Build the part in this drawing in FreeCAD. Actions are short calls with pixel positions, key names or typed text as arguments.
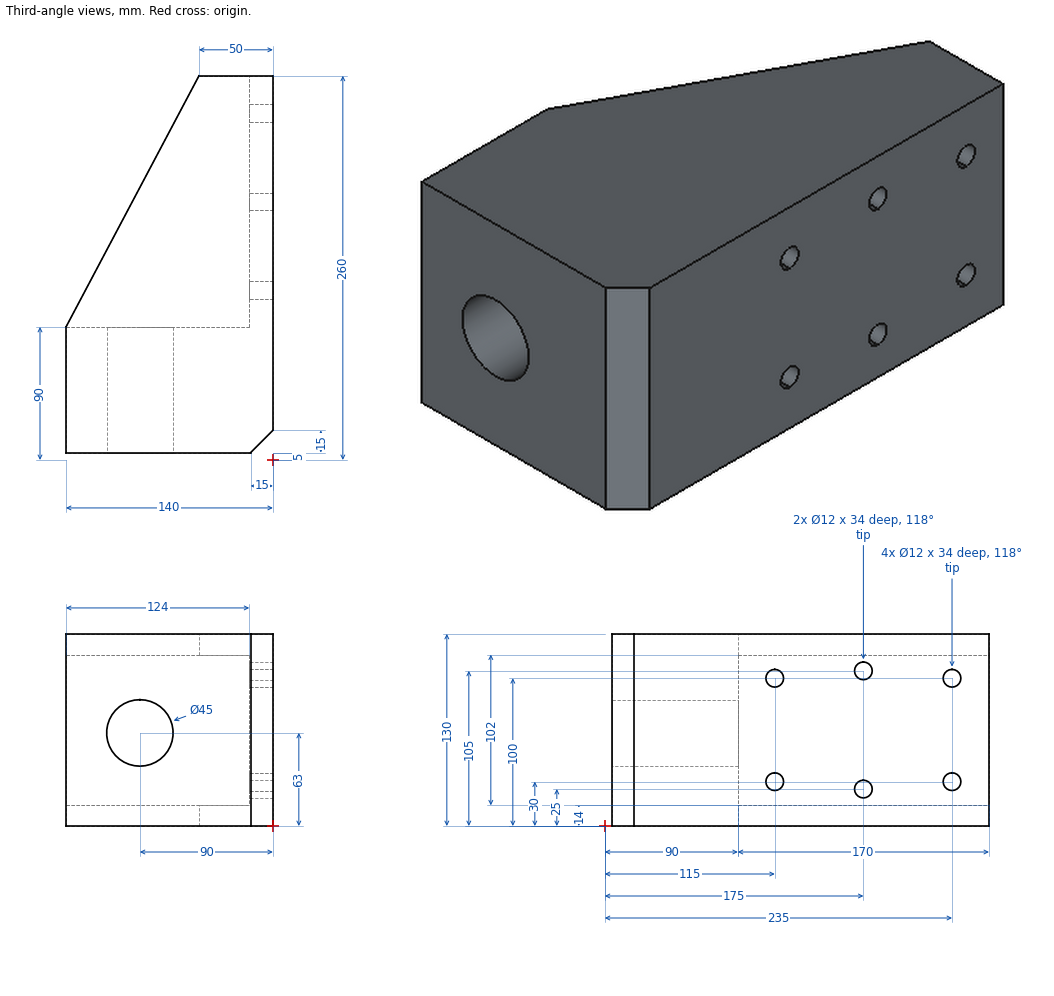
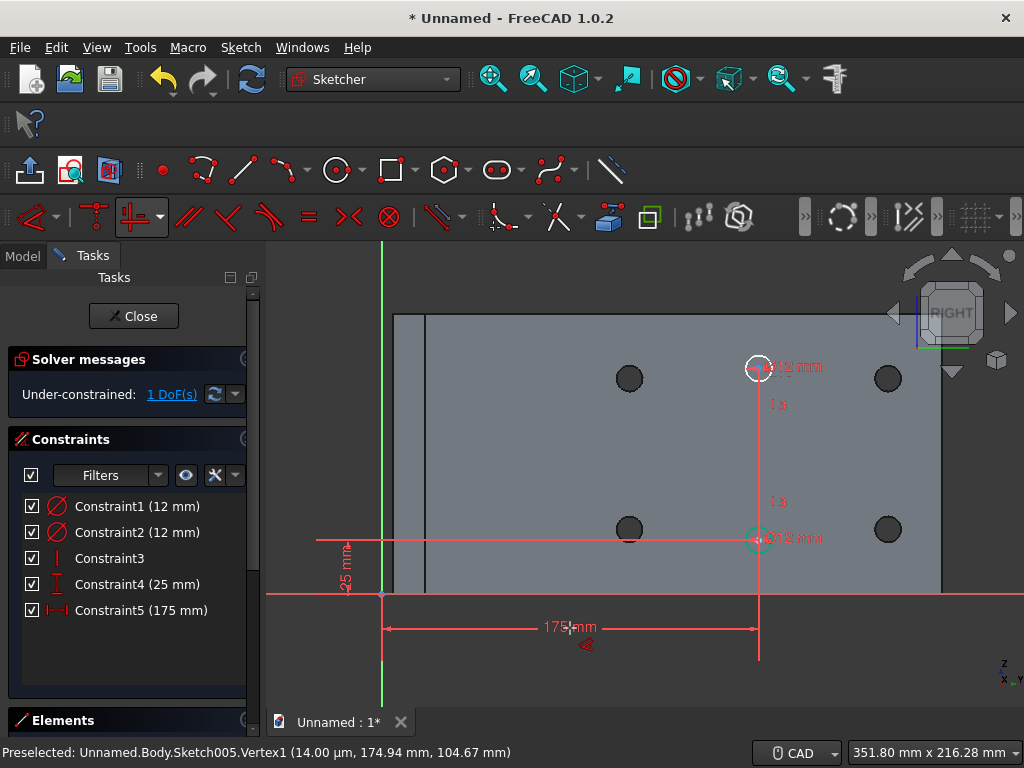
click(759, 369)
click(348, 481)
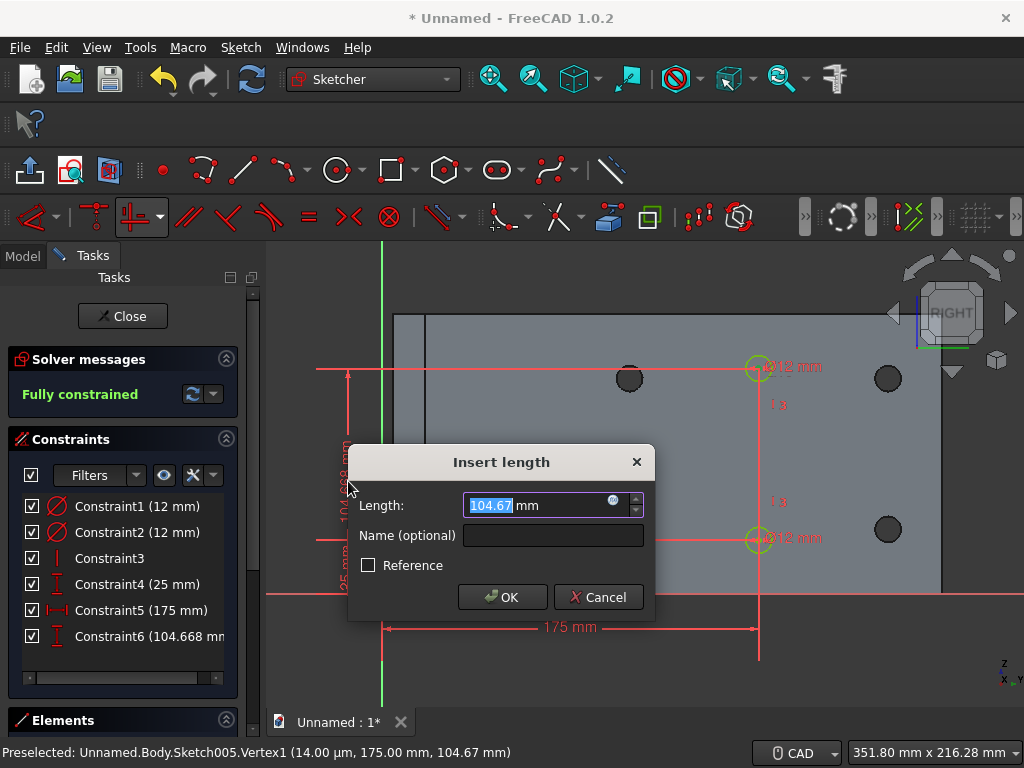
text(105)
key(Return)
key(Escape)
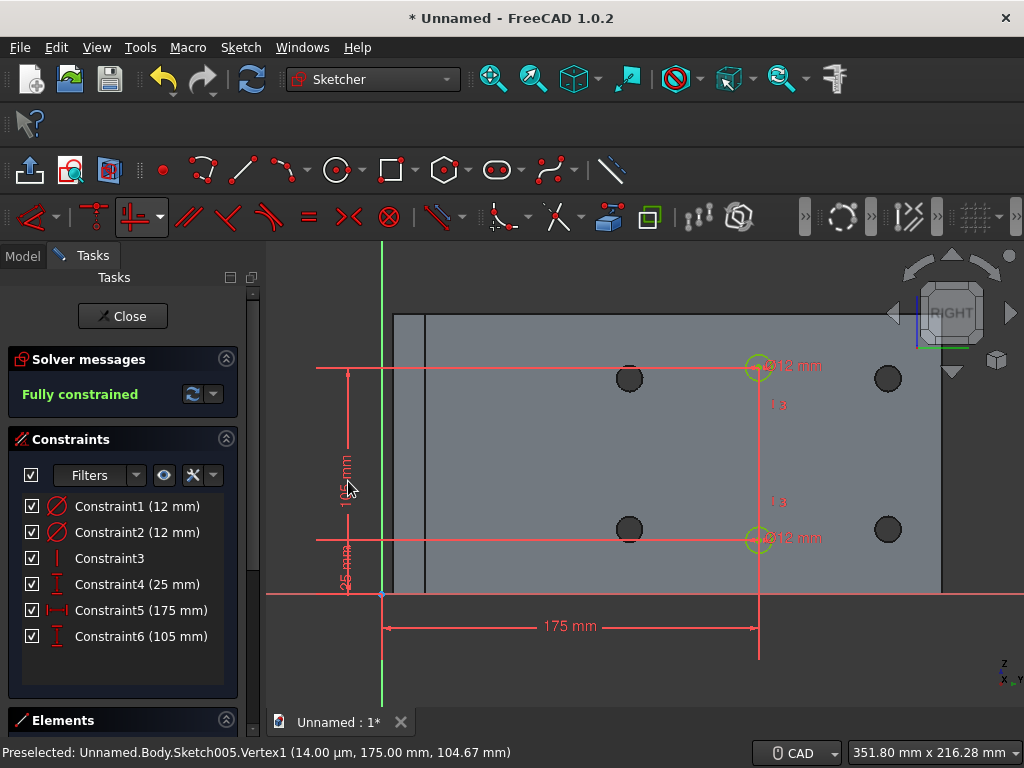
click(123, 316)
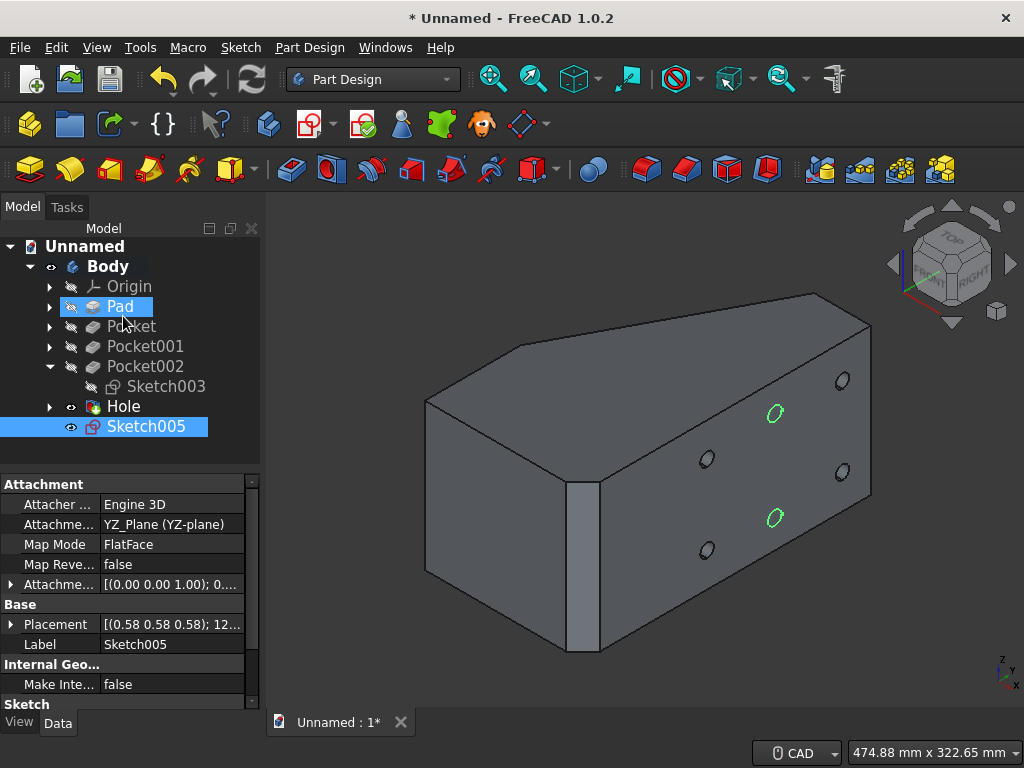
click(332, 170)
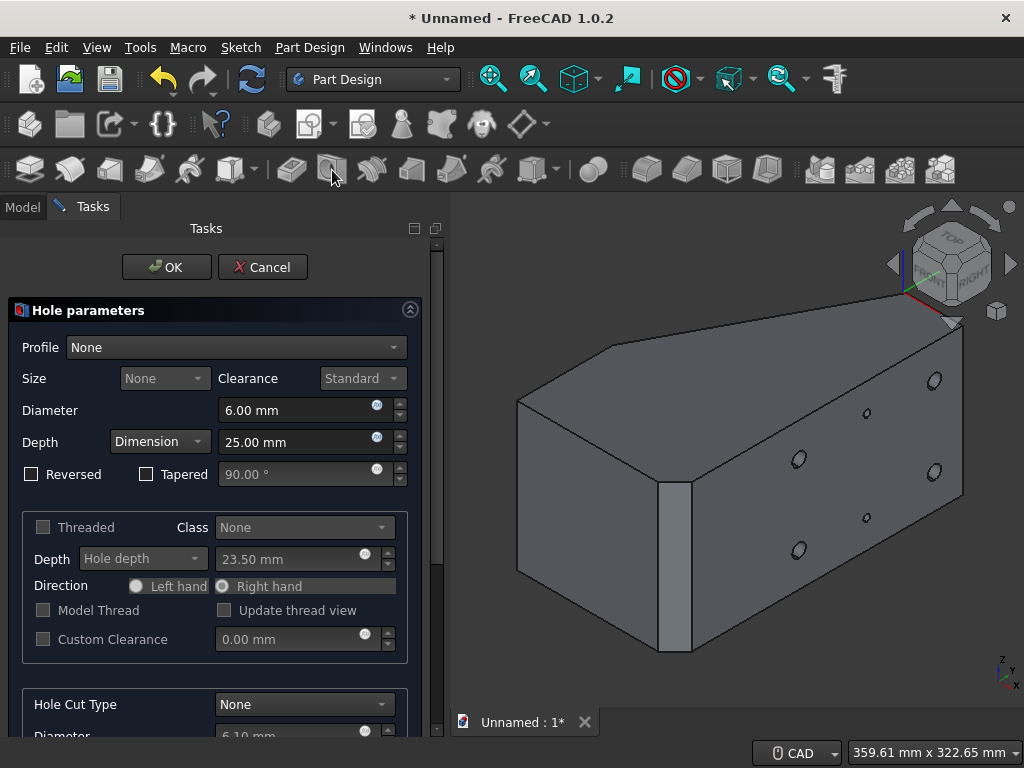
triple_click(305, 410)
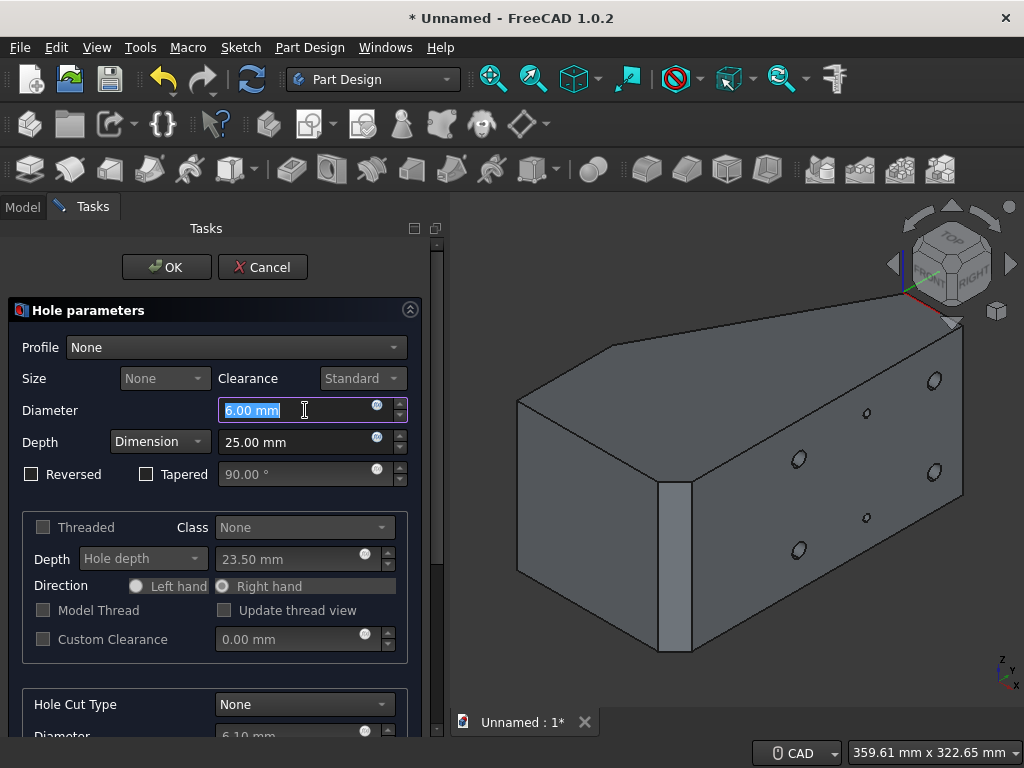
text(12)
key(Tab)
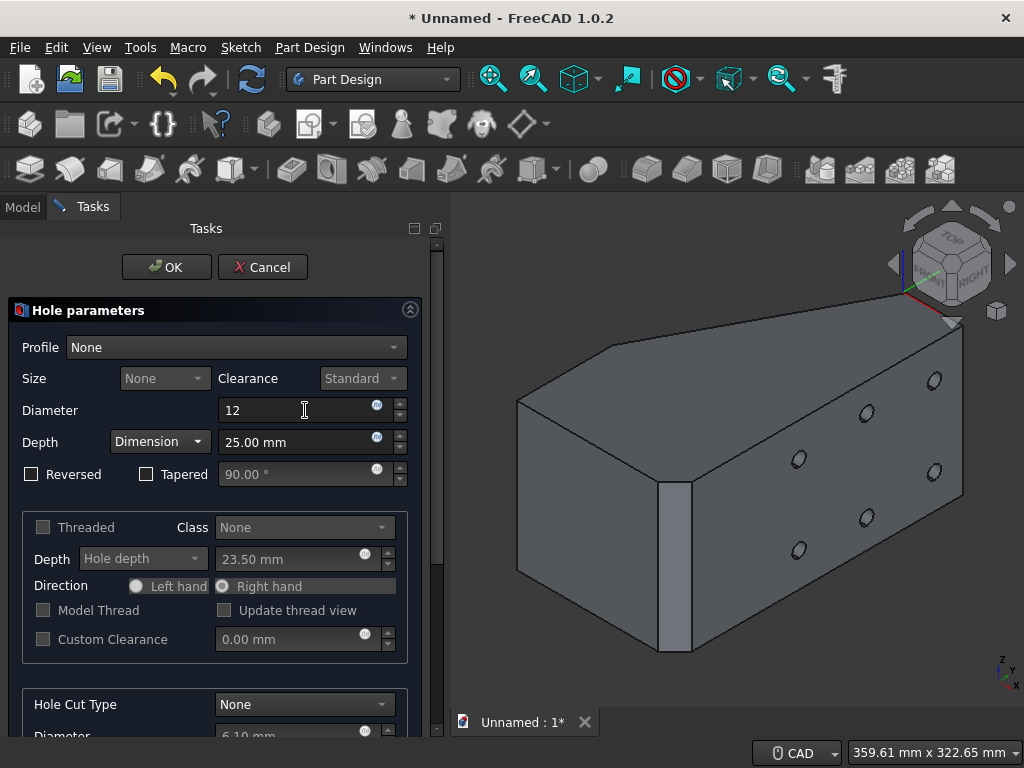
triple_click(305, 442)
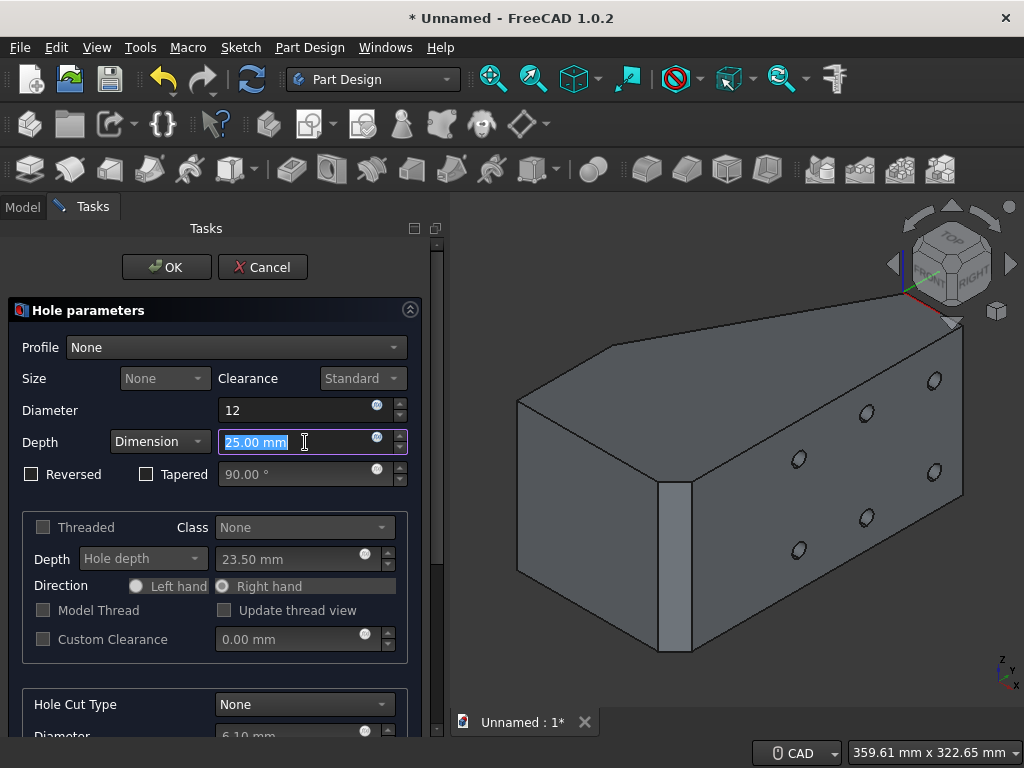
text(34)
key(Tab)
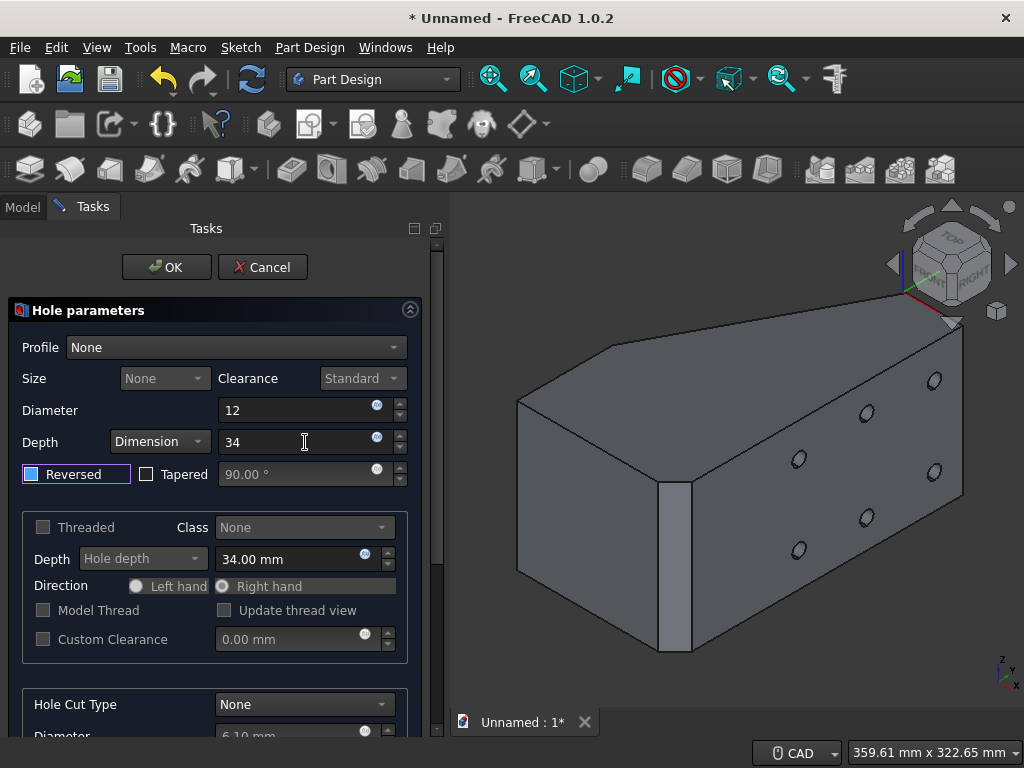
click(167, 267)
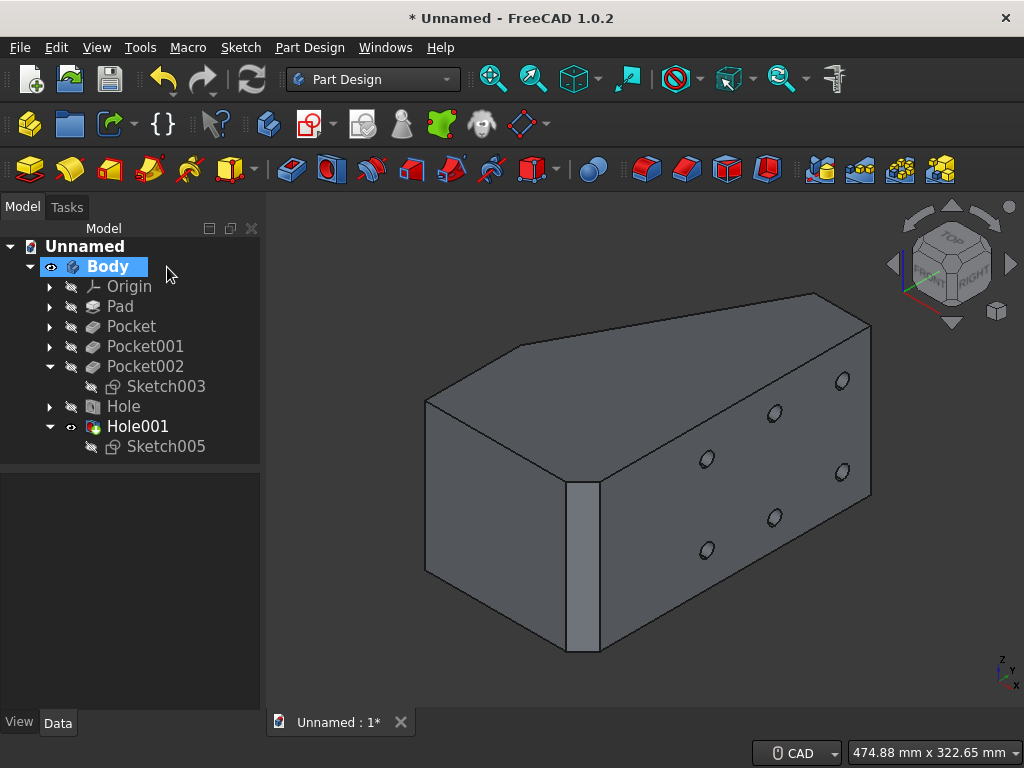
click(495, 525)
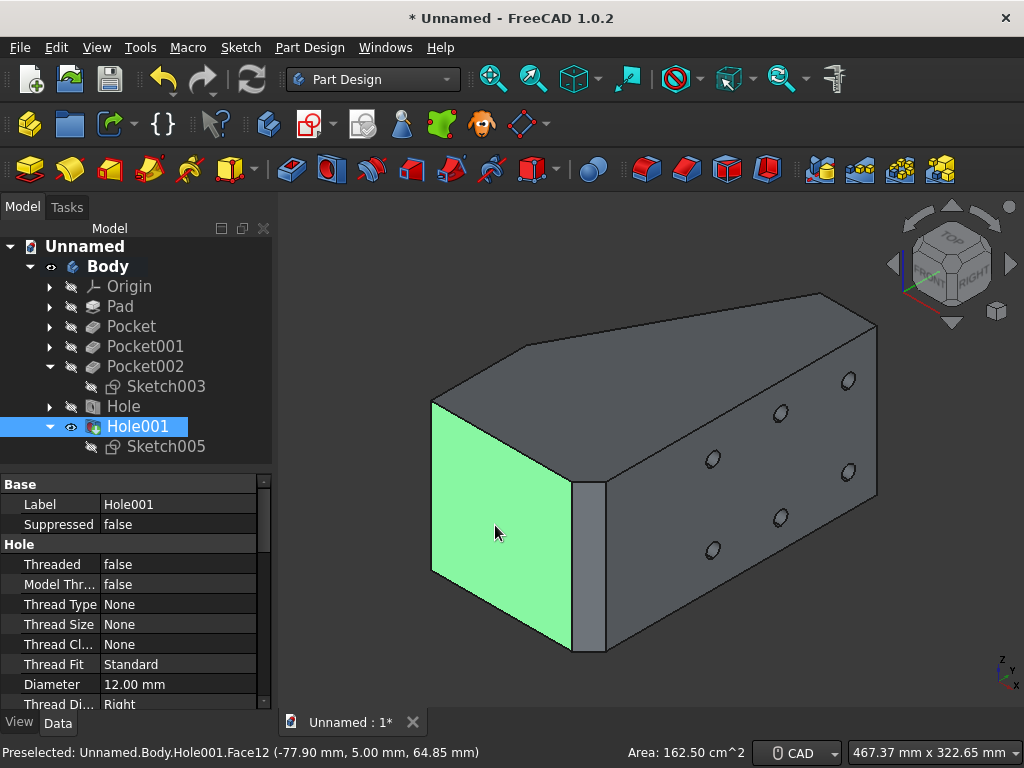
click(310, 124)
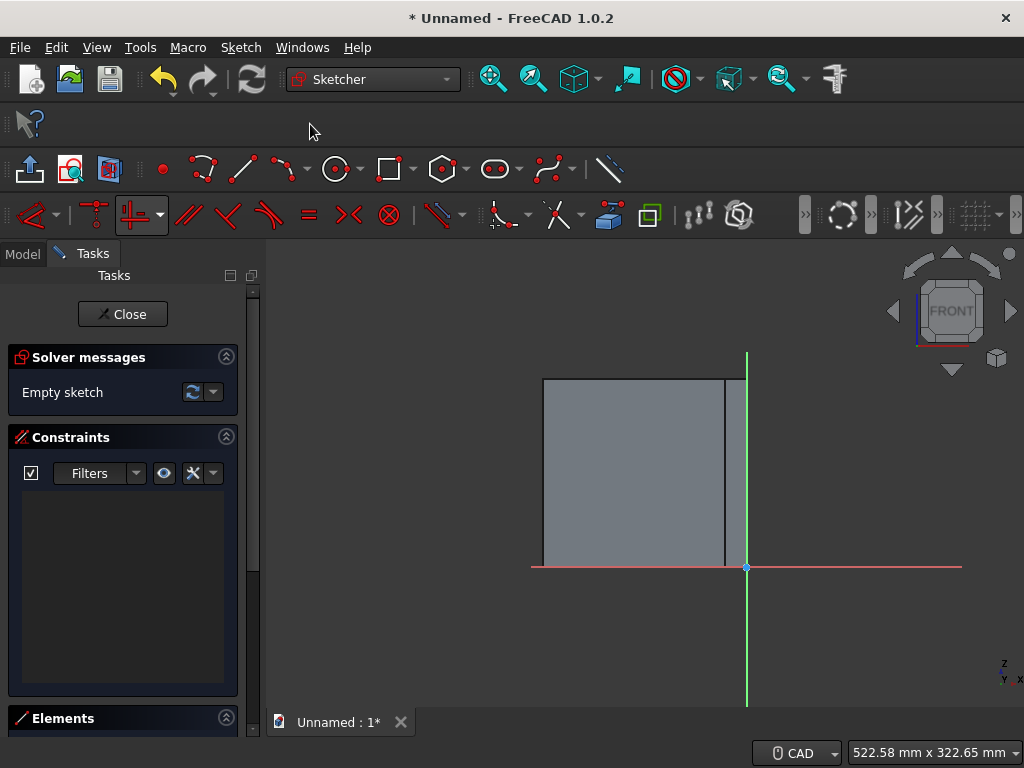
scroll(629, 477, up, 7)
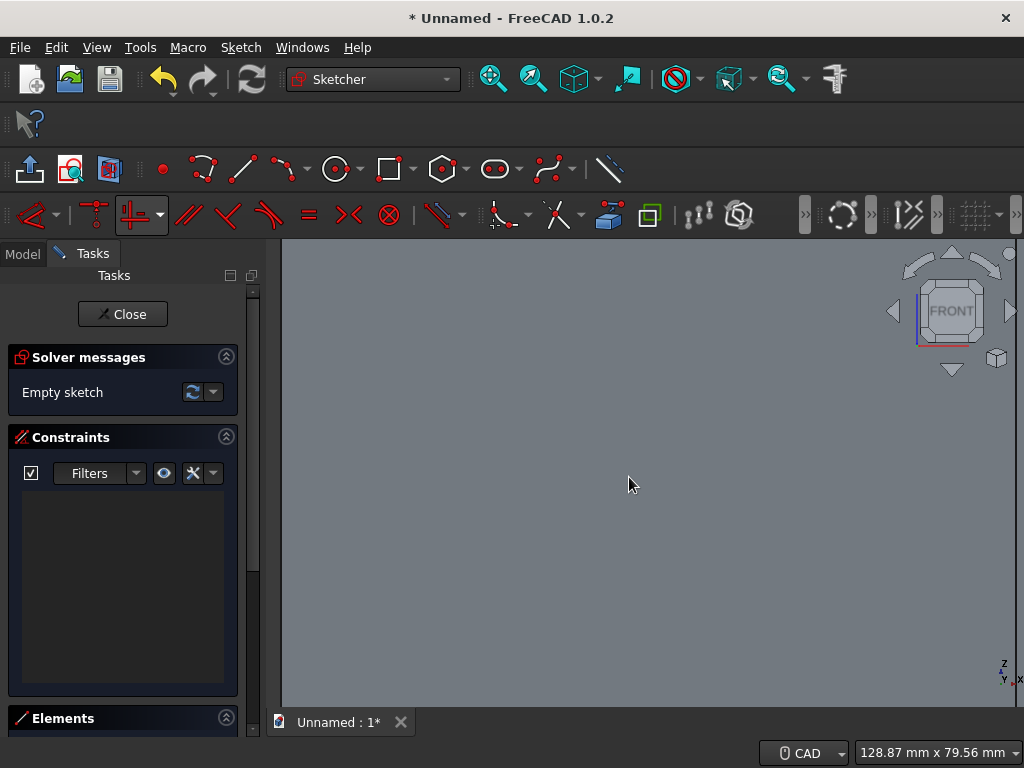
click(336, 170)